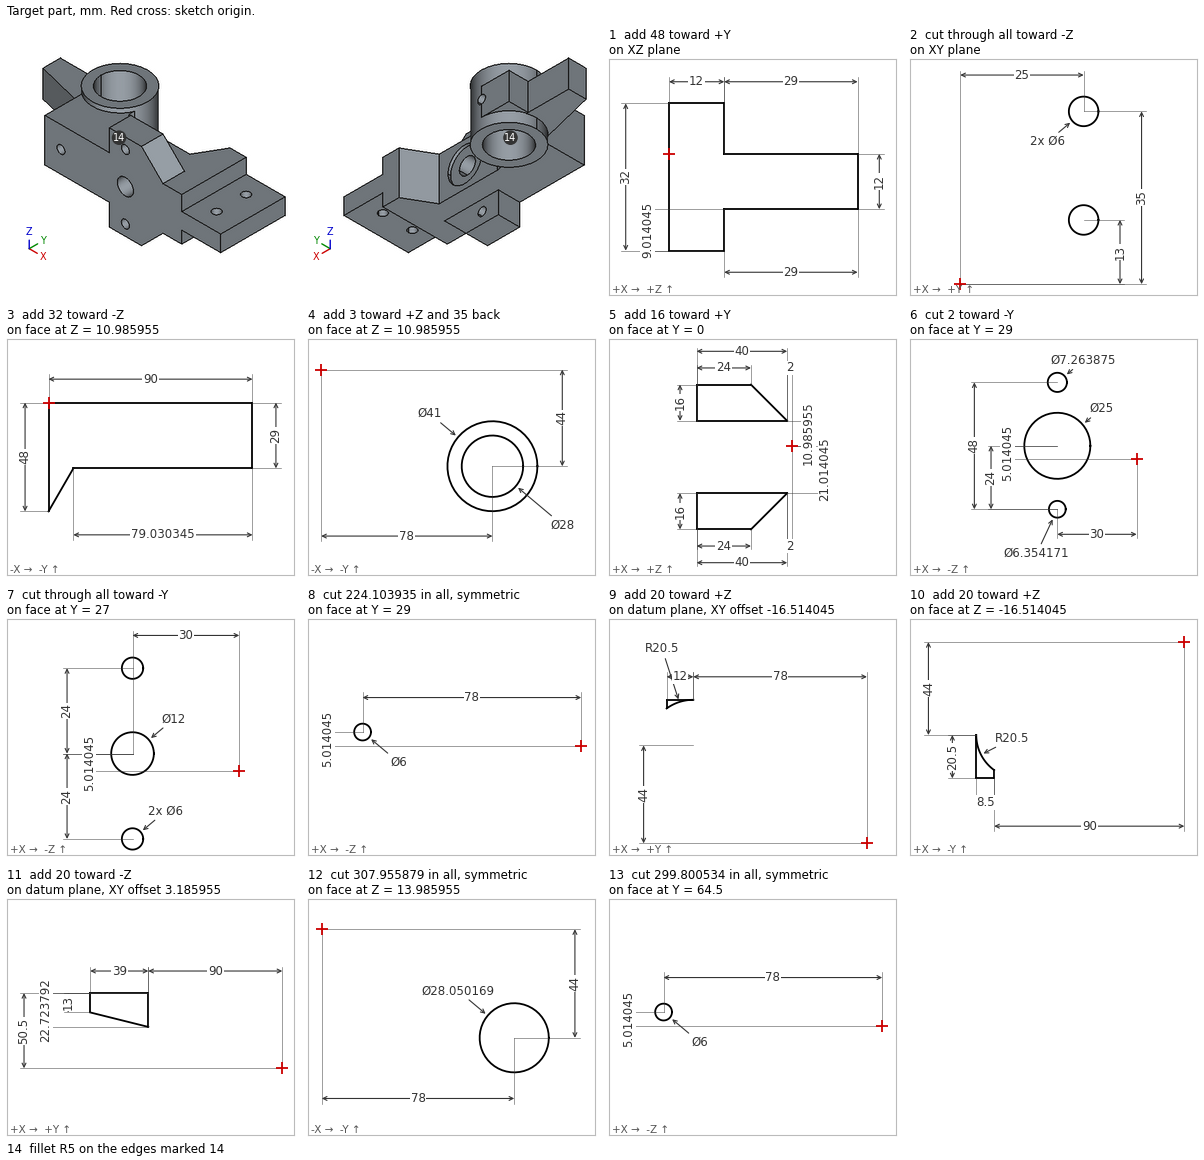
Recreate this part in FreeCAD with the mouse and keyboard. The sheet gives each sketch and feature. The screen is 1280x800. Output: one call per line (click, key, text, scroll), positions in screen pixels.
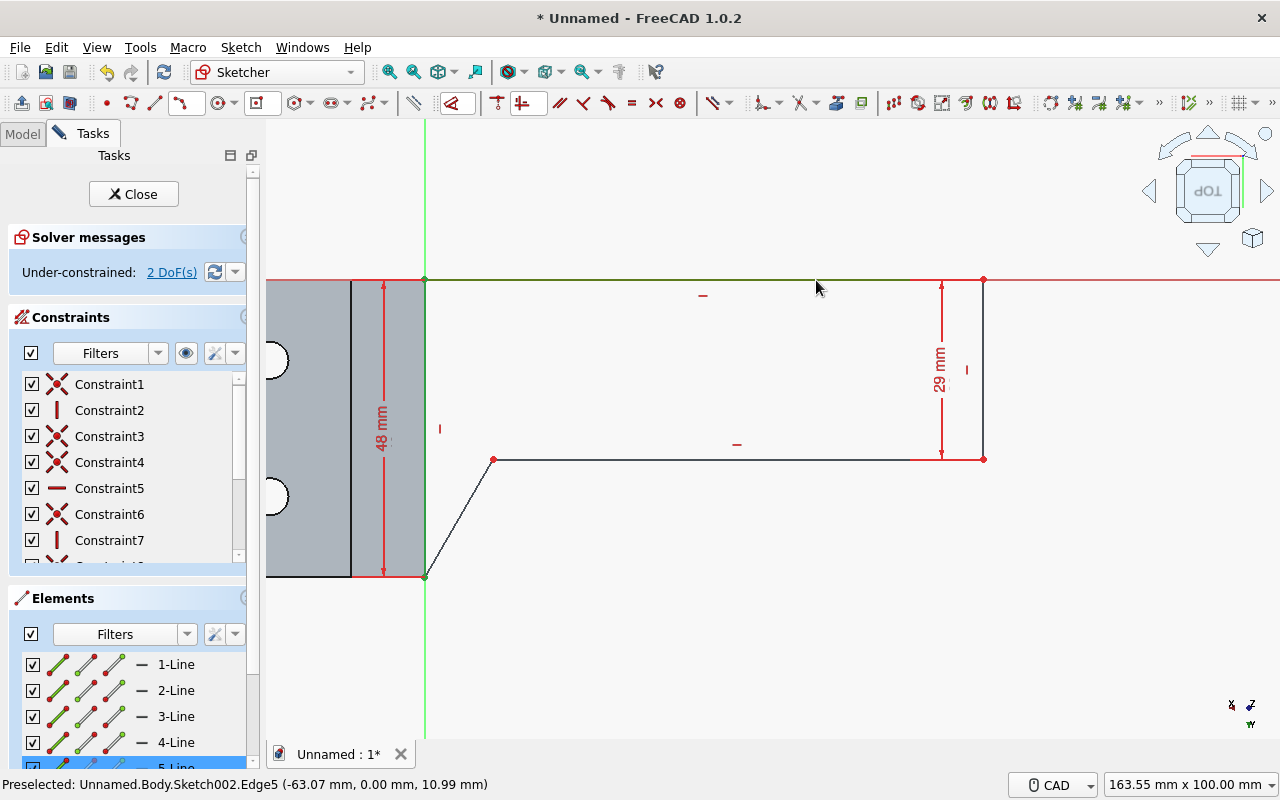
key(l)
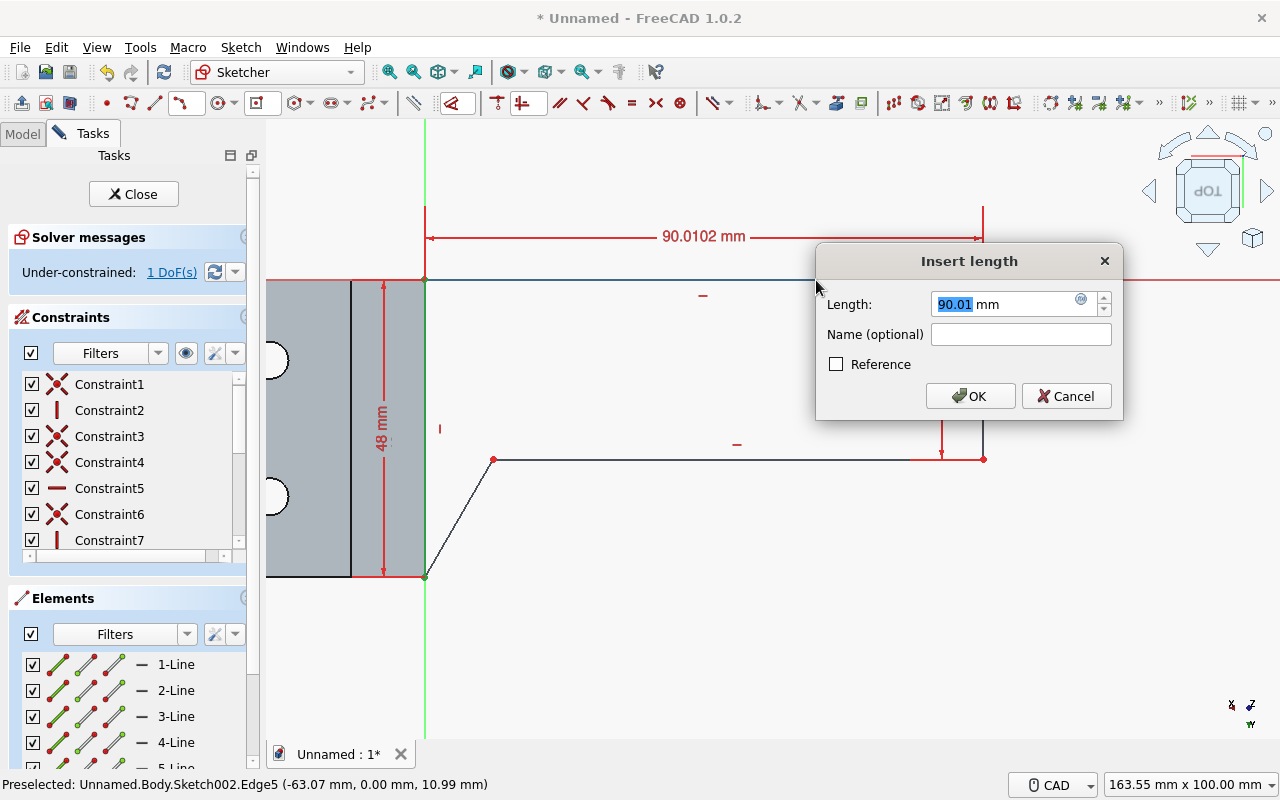
text(90)
key(Return)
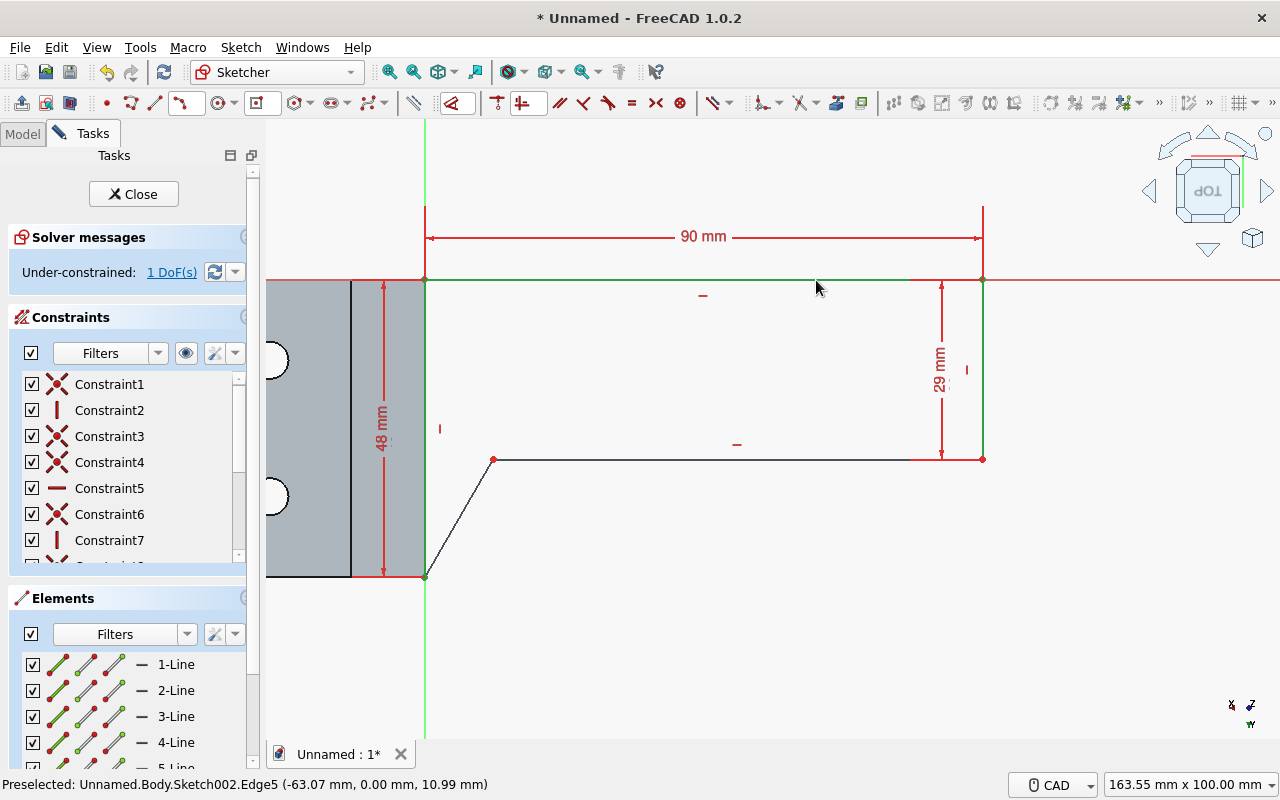
click(640, 460)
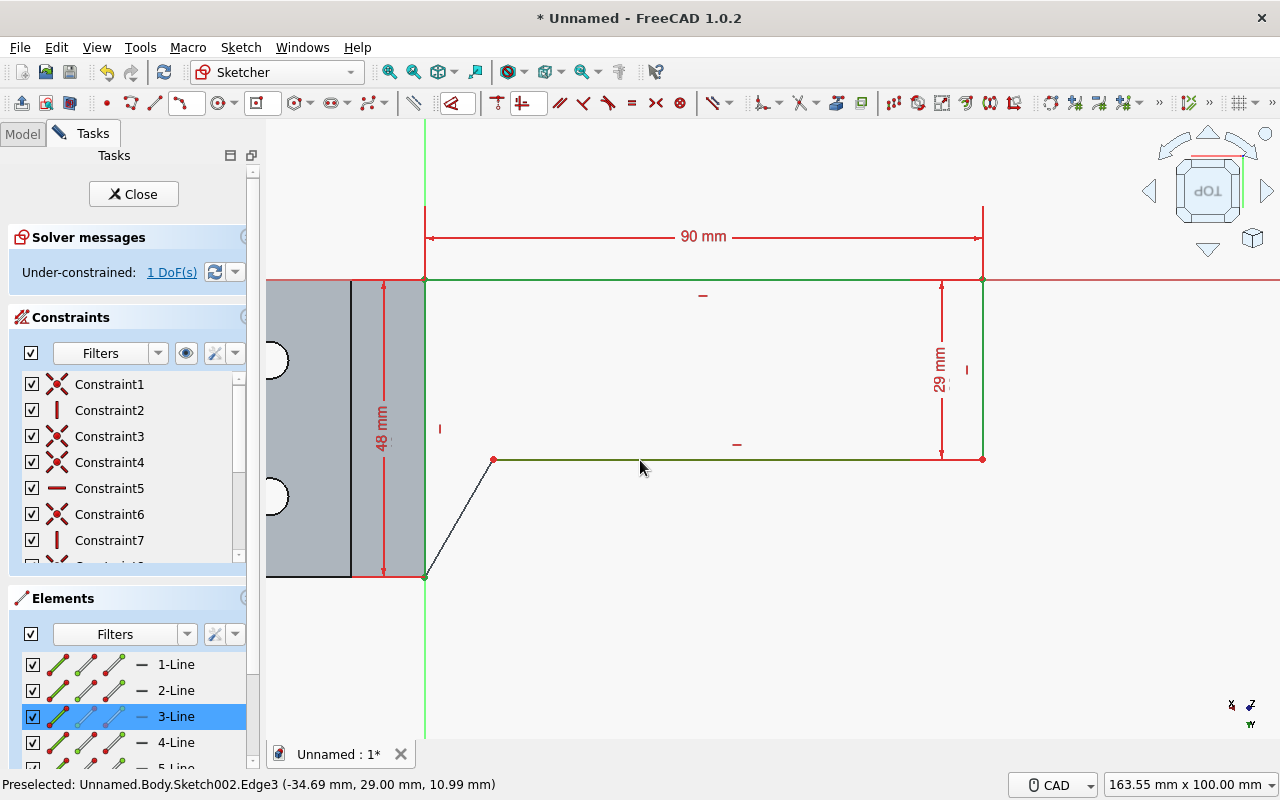
key(l)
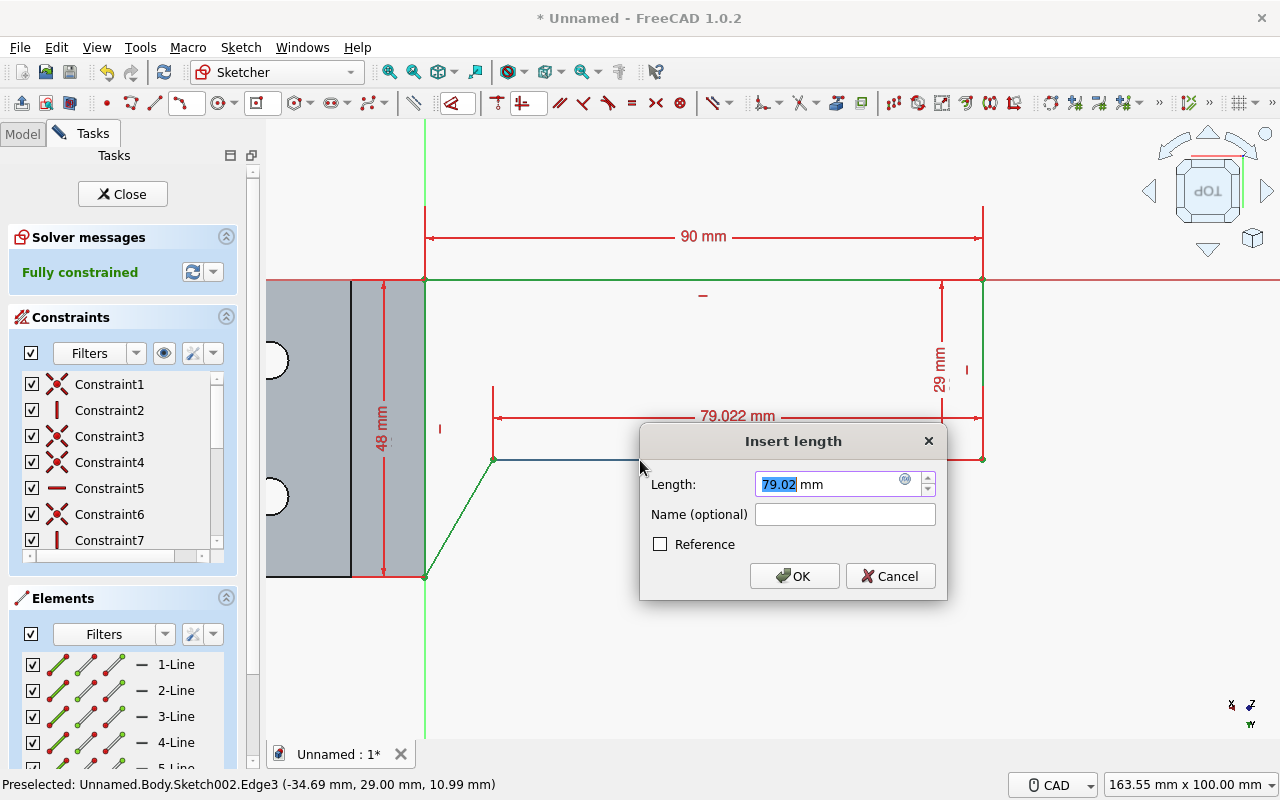
text(79.030345)
key(Return)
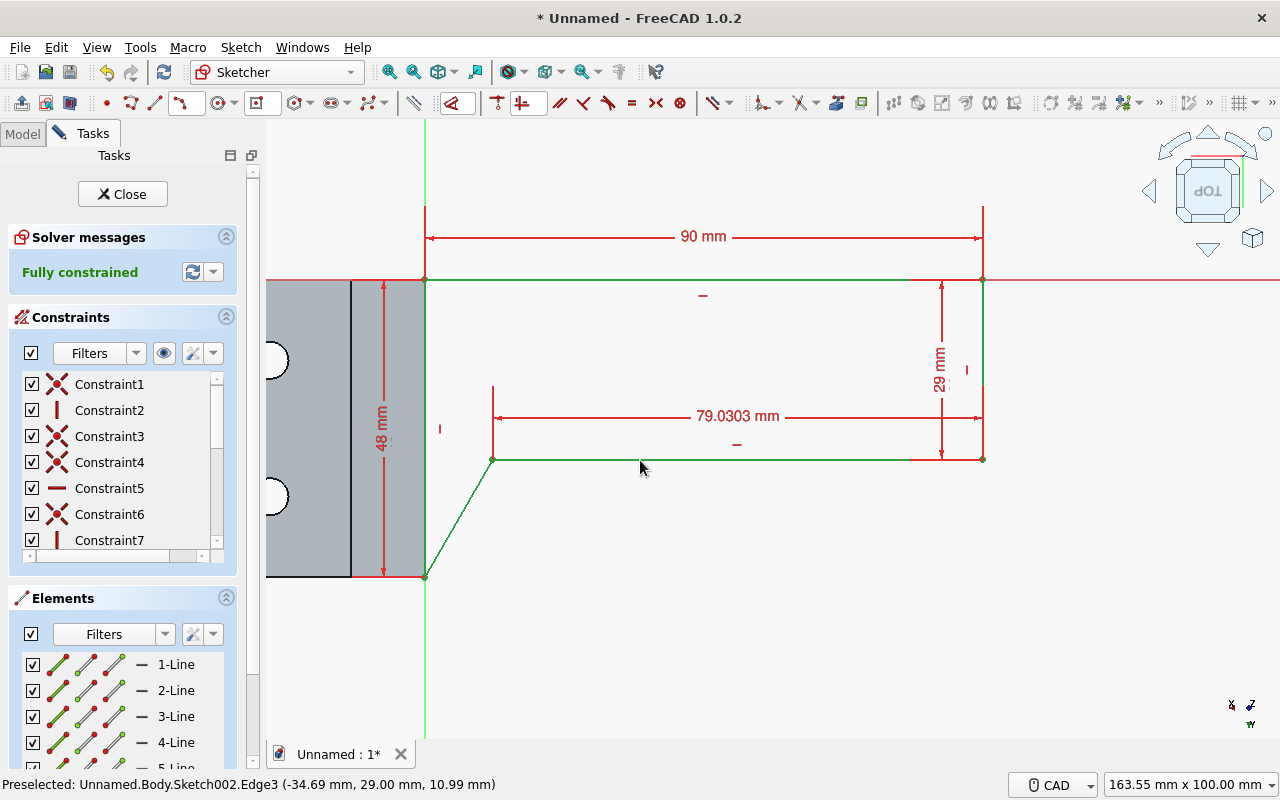
click(123, 194)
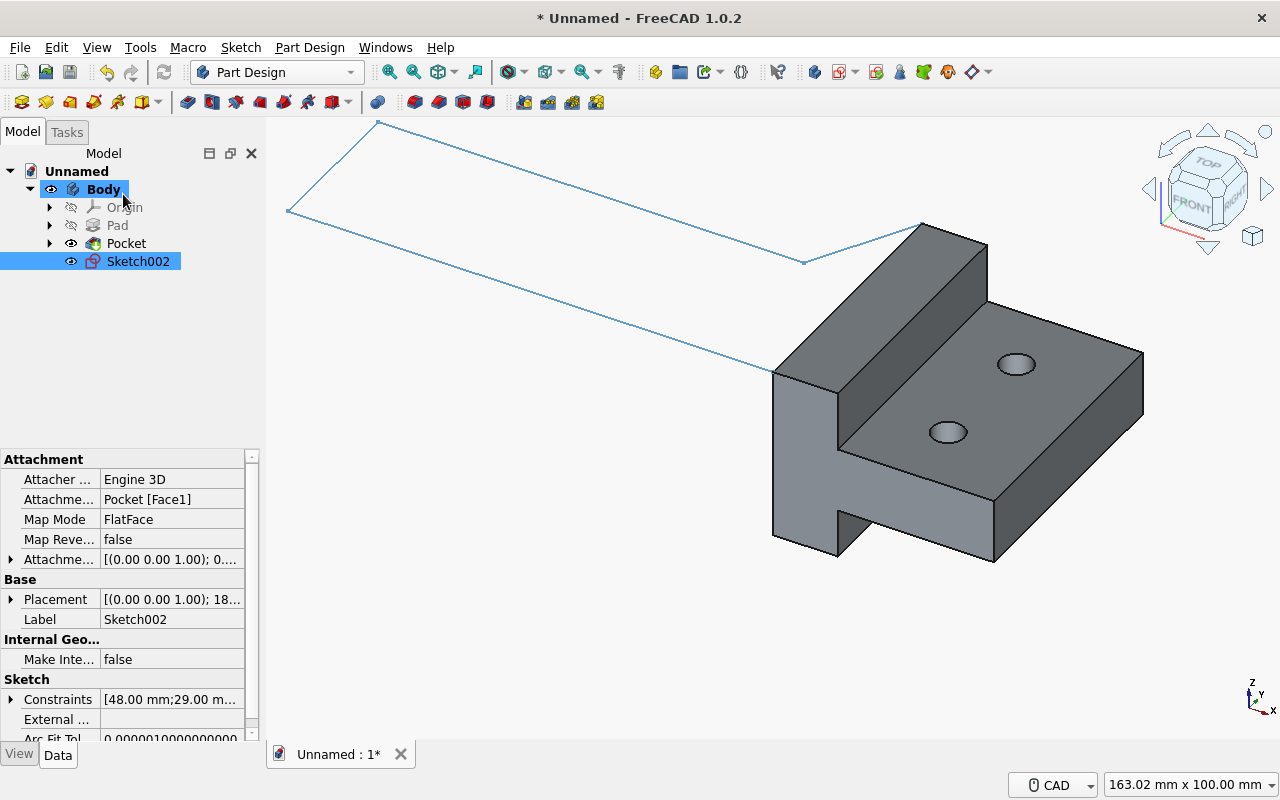
click(22, 102)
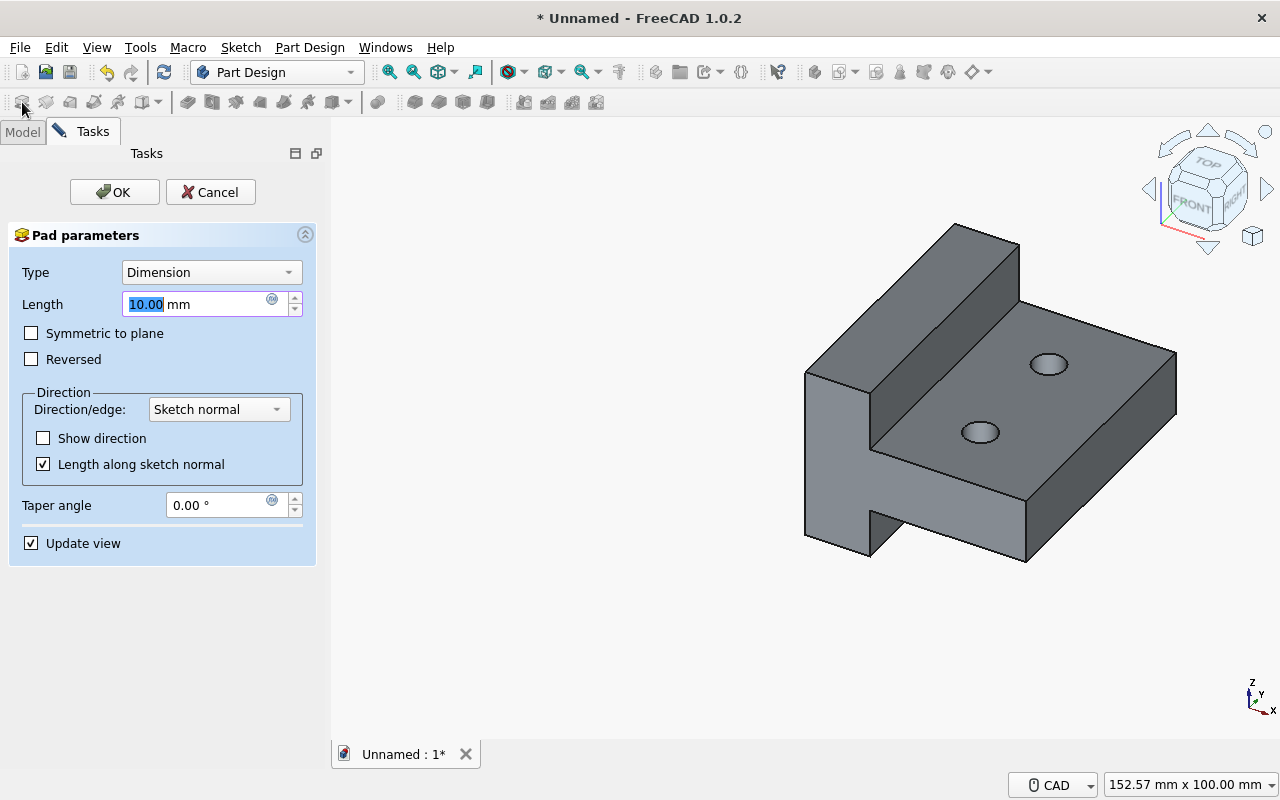
text(32)
key(Tab)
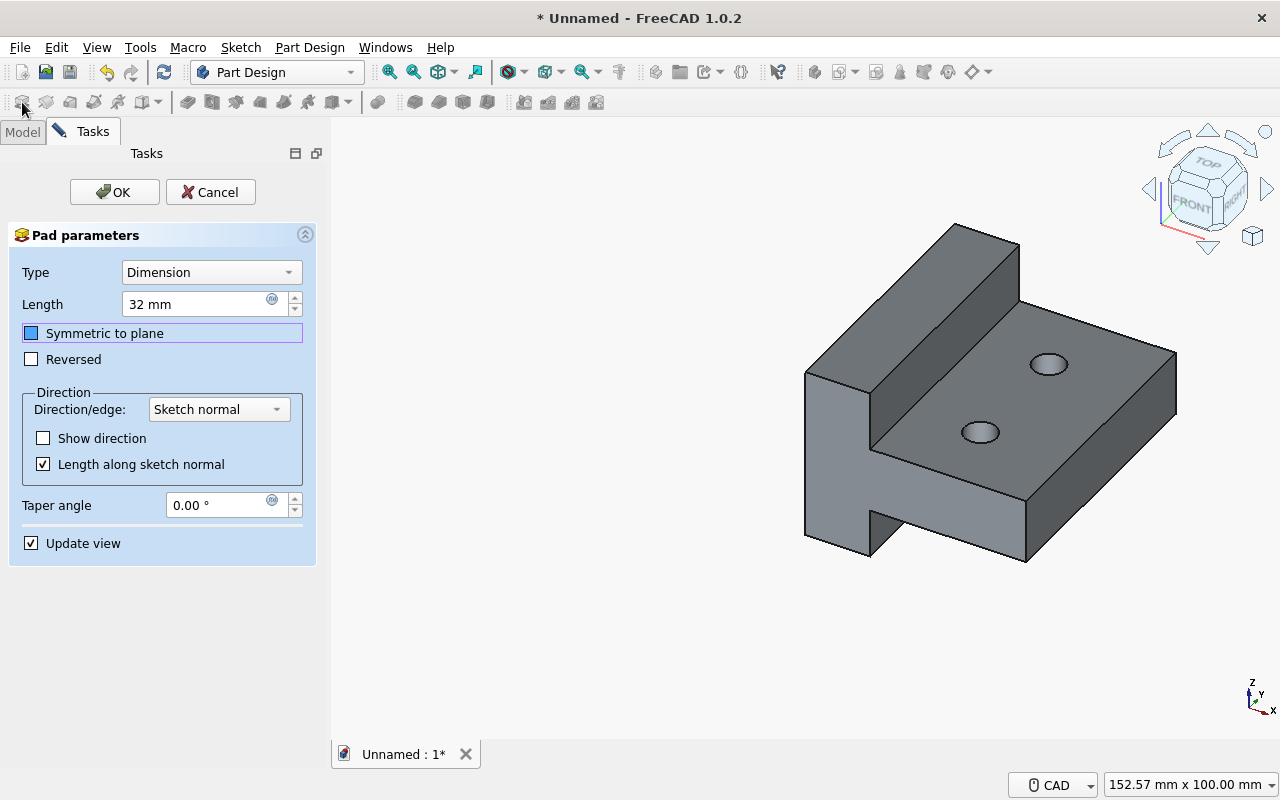
click(30, 359)